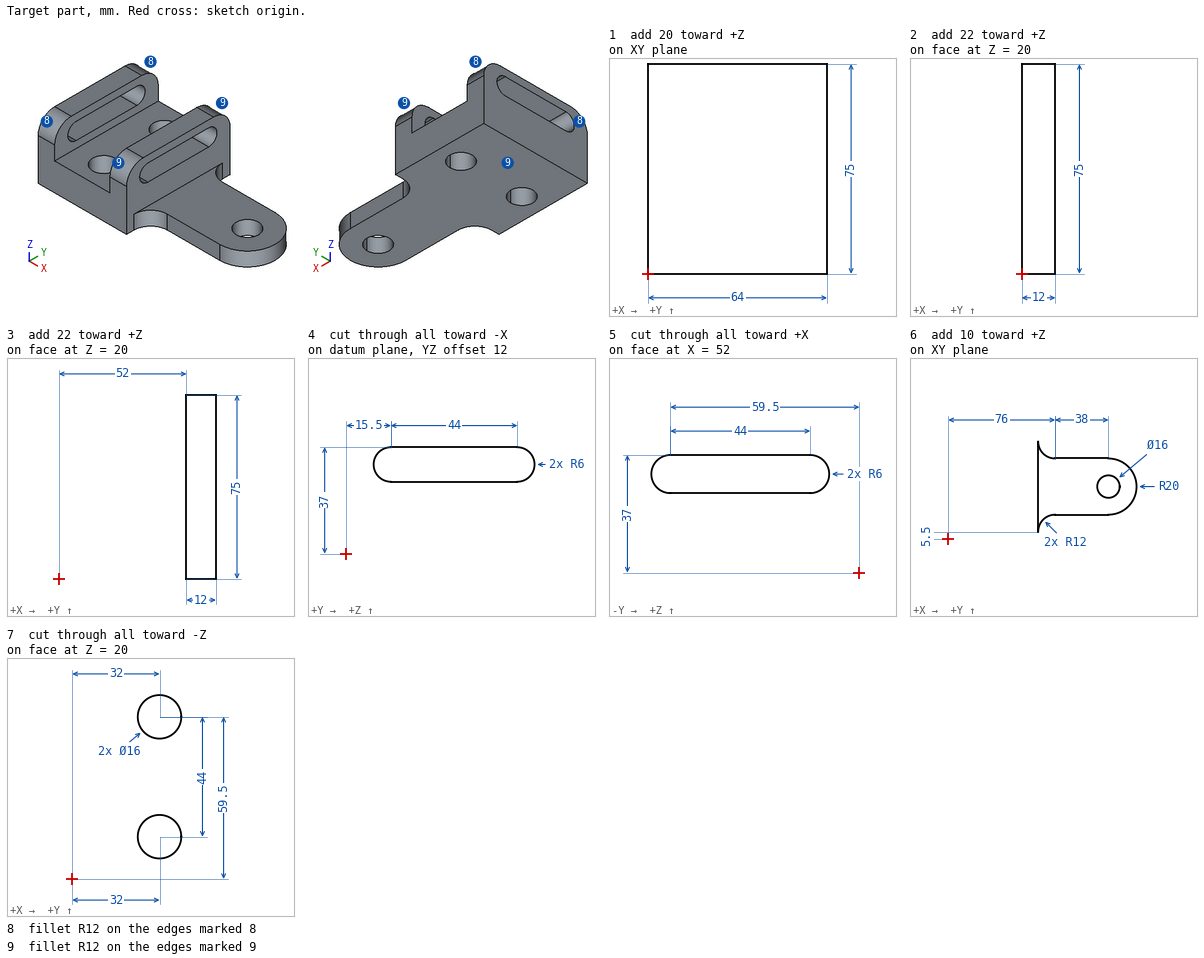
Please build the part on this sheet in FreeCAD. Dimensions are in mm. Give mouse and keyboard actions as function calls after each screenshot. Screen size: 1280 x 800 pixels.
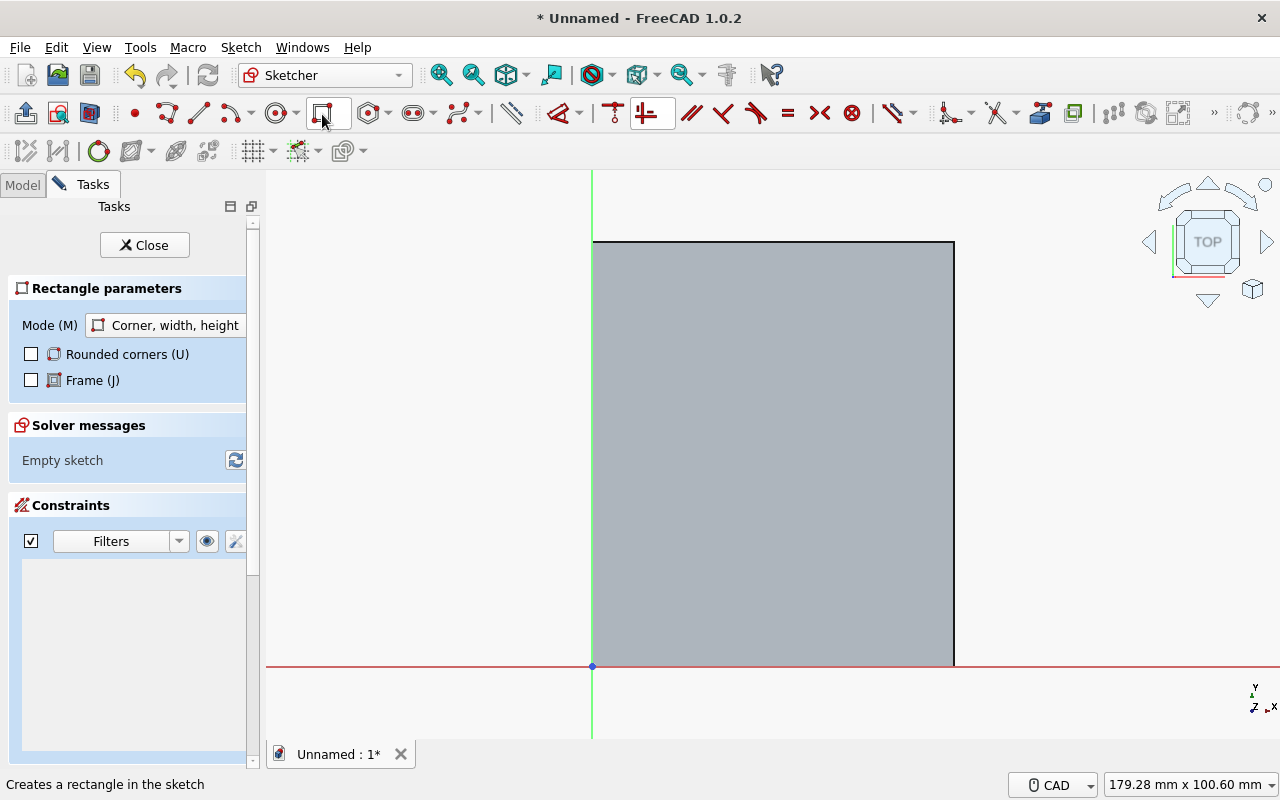
click(592, 667)
click(660, 242)
key(Escape)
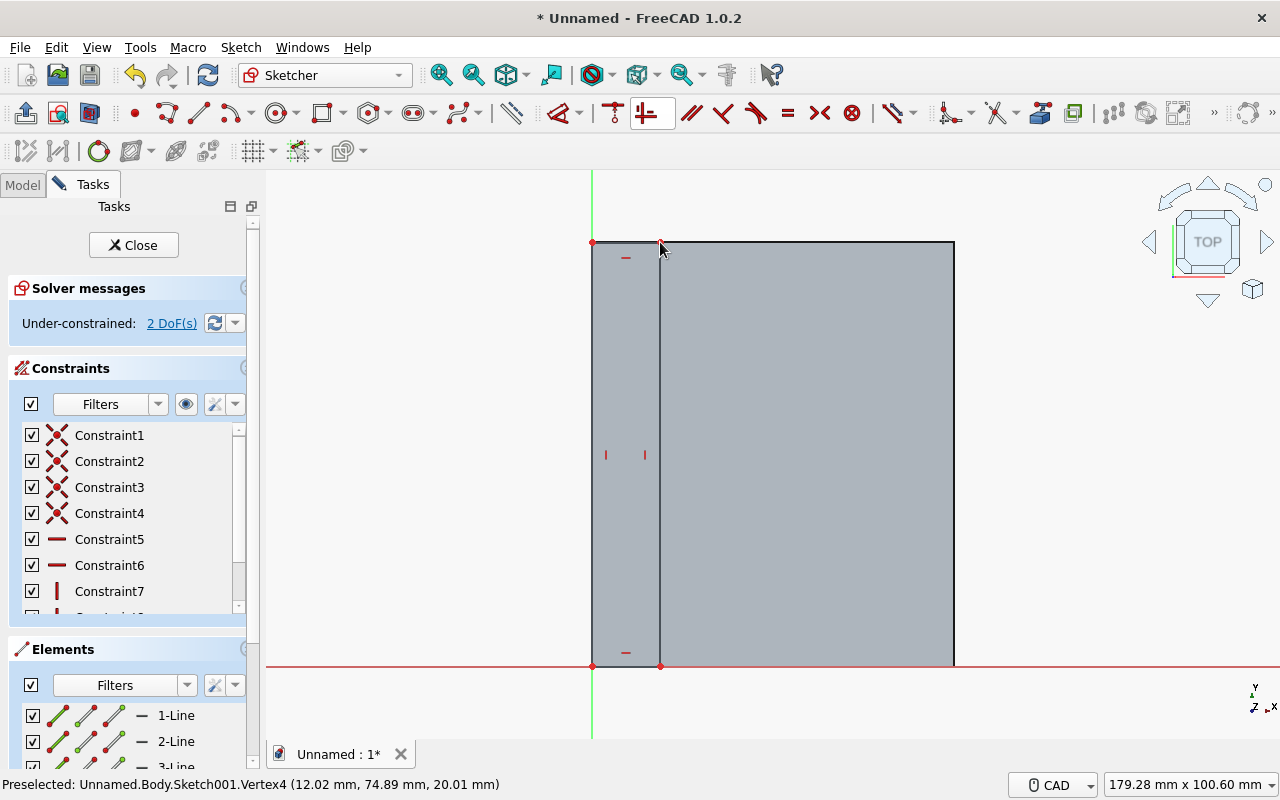
click(558, 114)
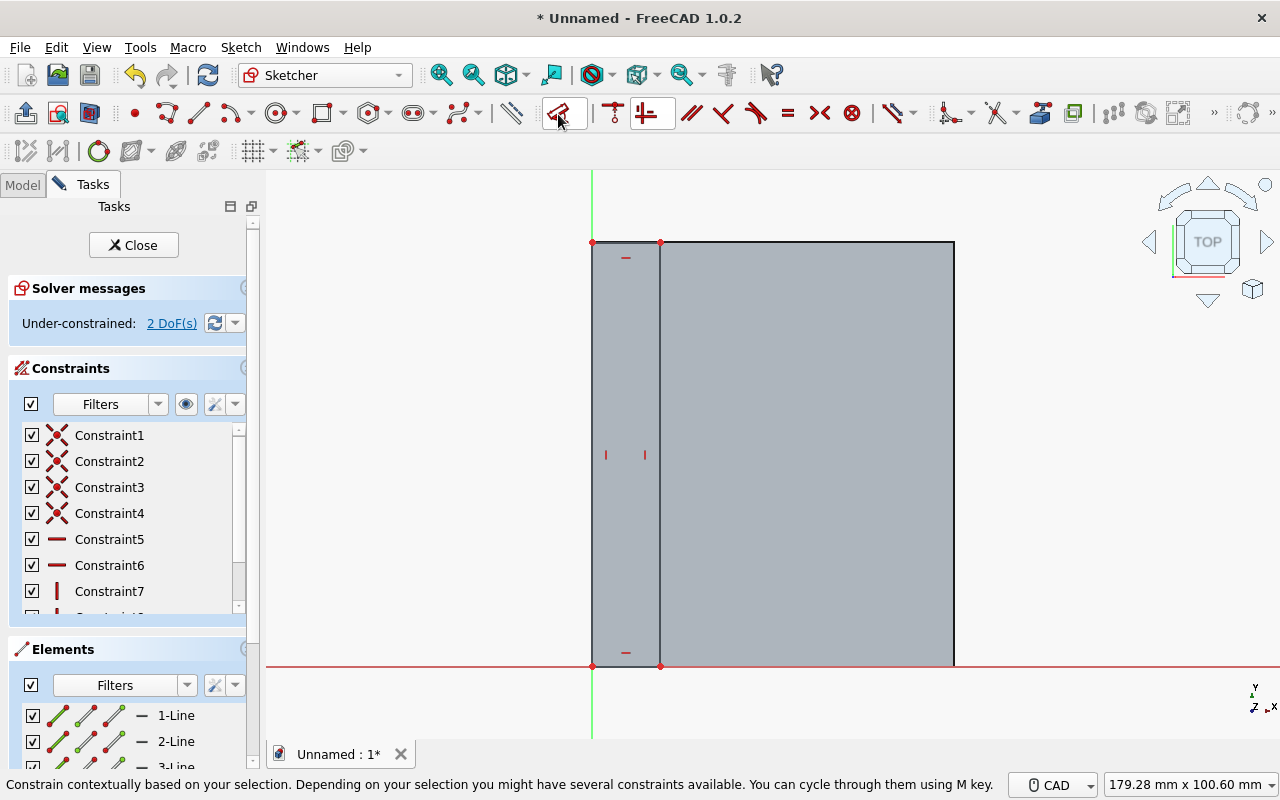
click(612, 667)
click(626, 701)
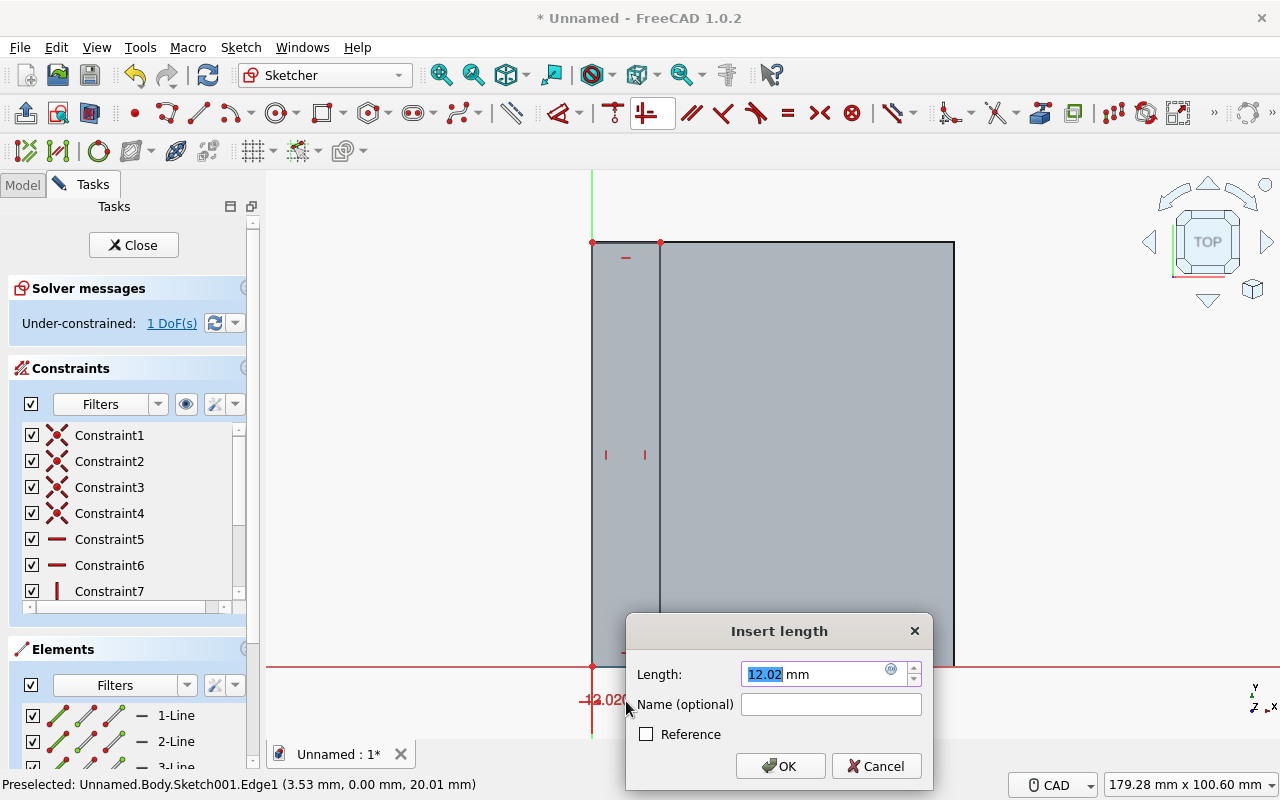
text(12)
key(Return)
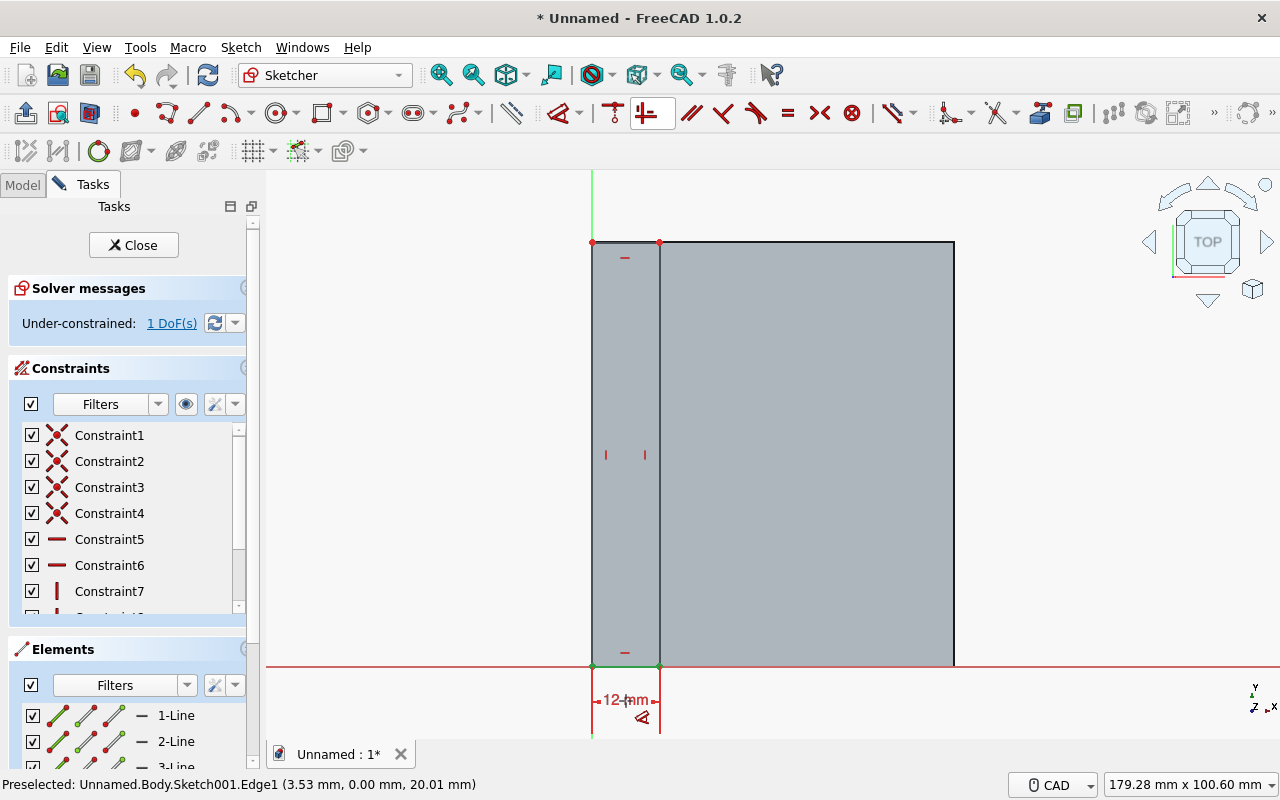
click(660, 540)
click(694, 455)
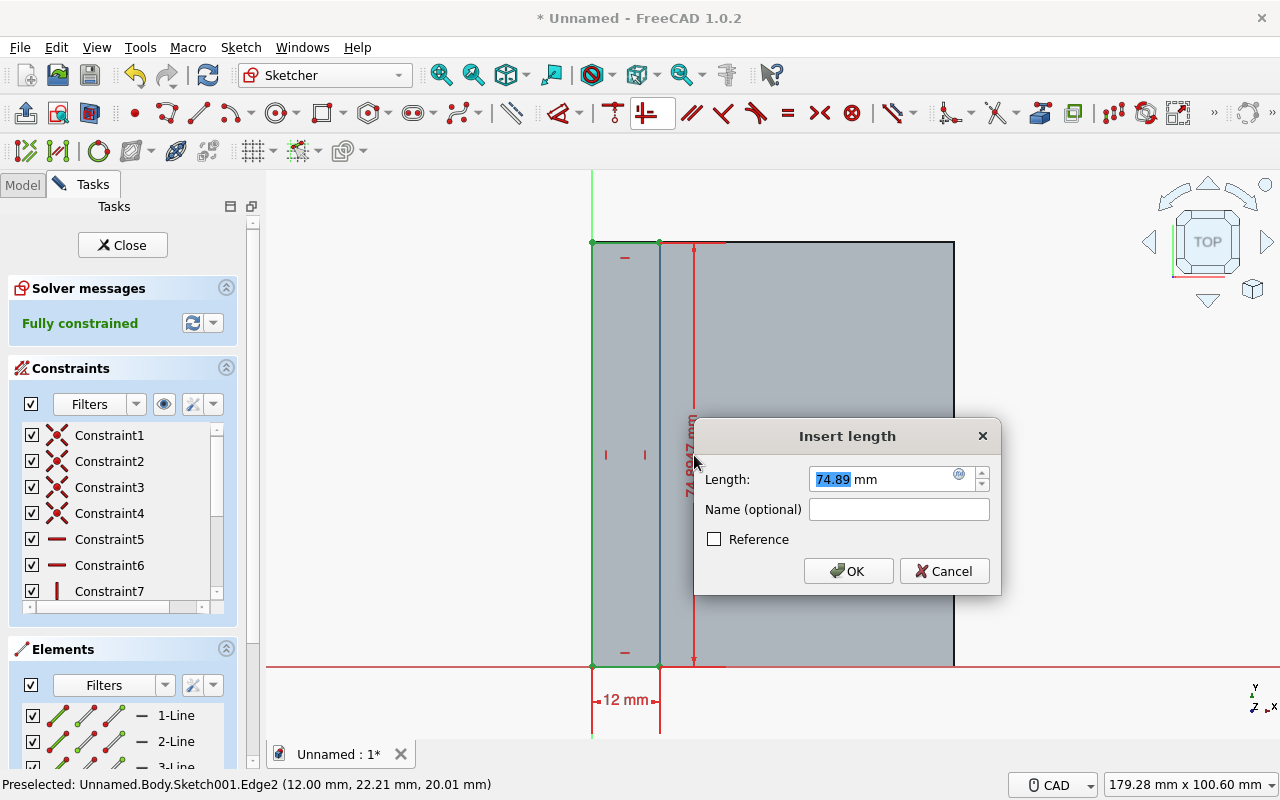
text(75)
key(Return)
key(Escape)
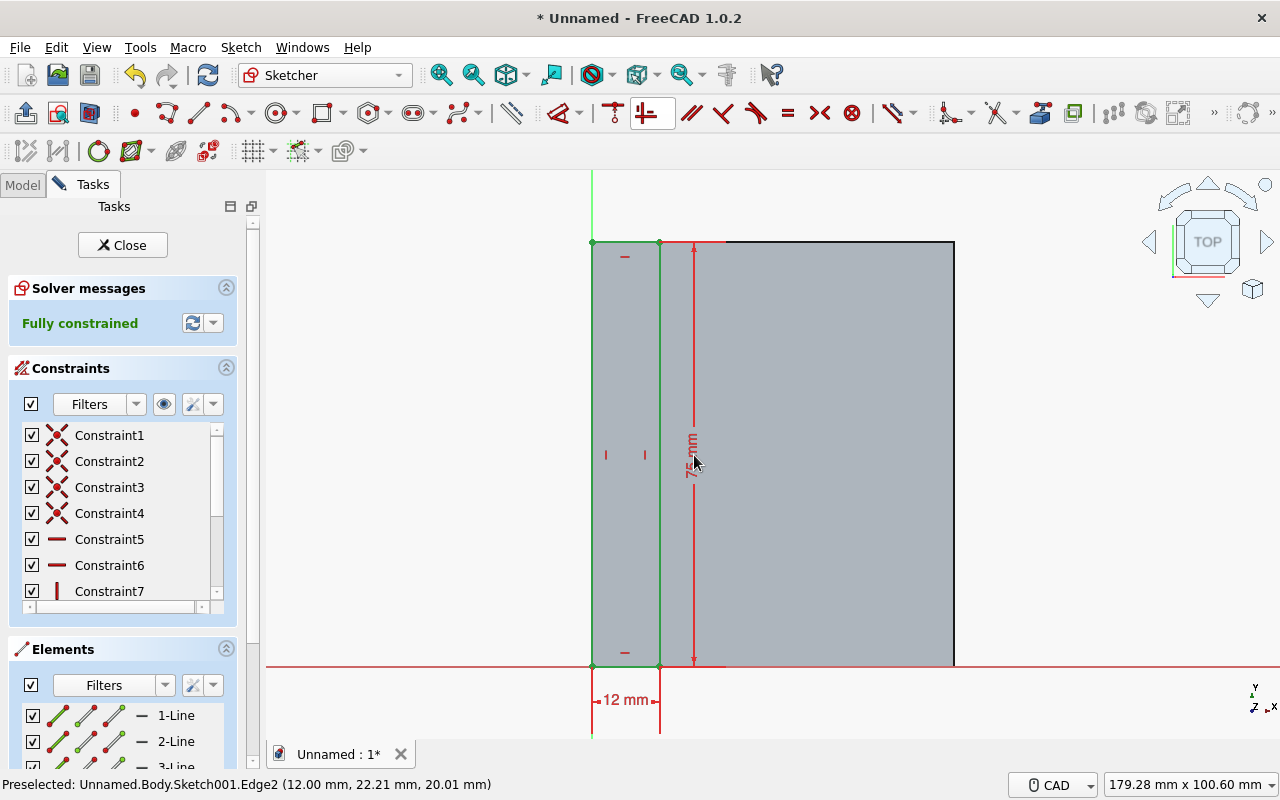
click(123, 245)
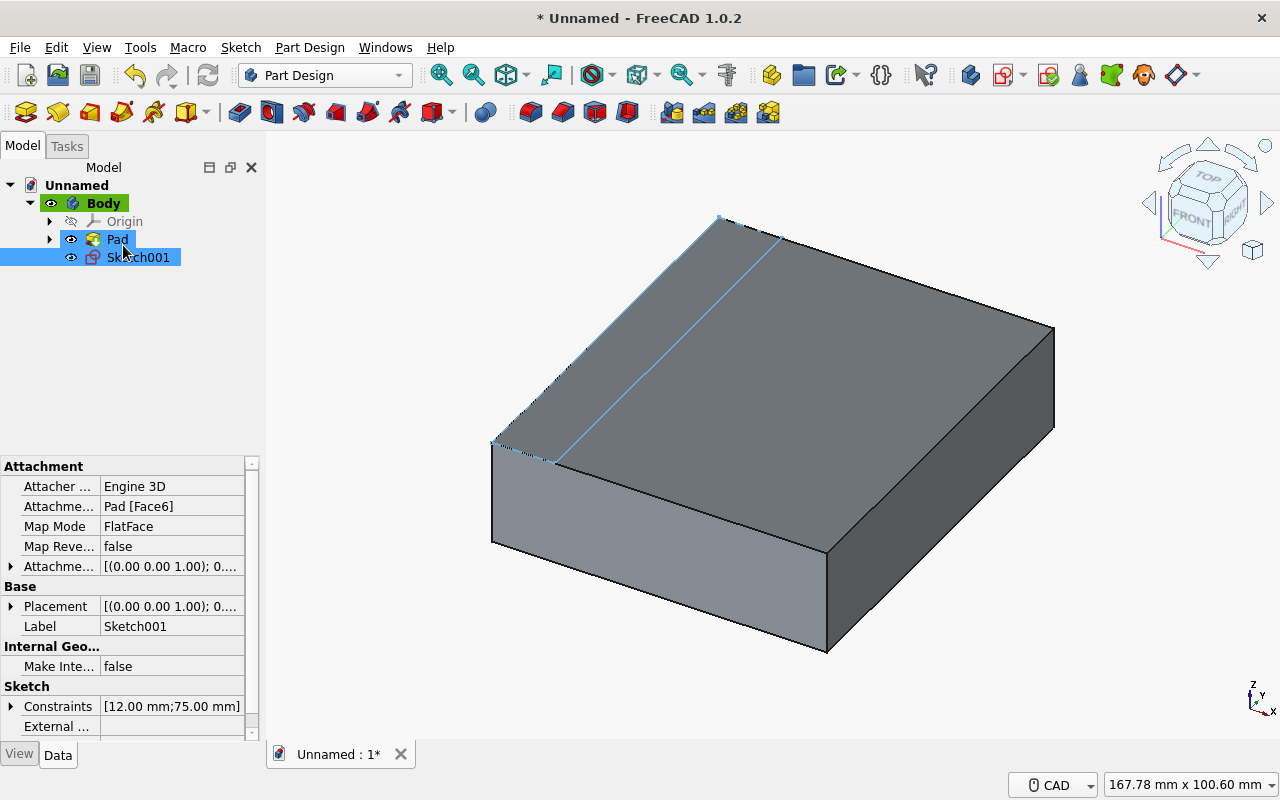
click(26, 112)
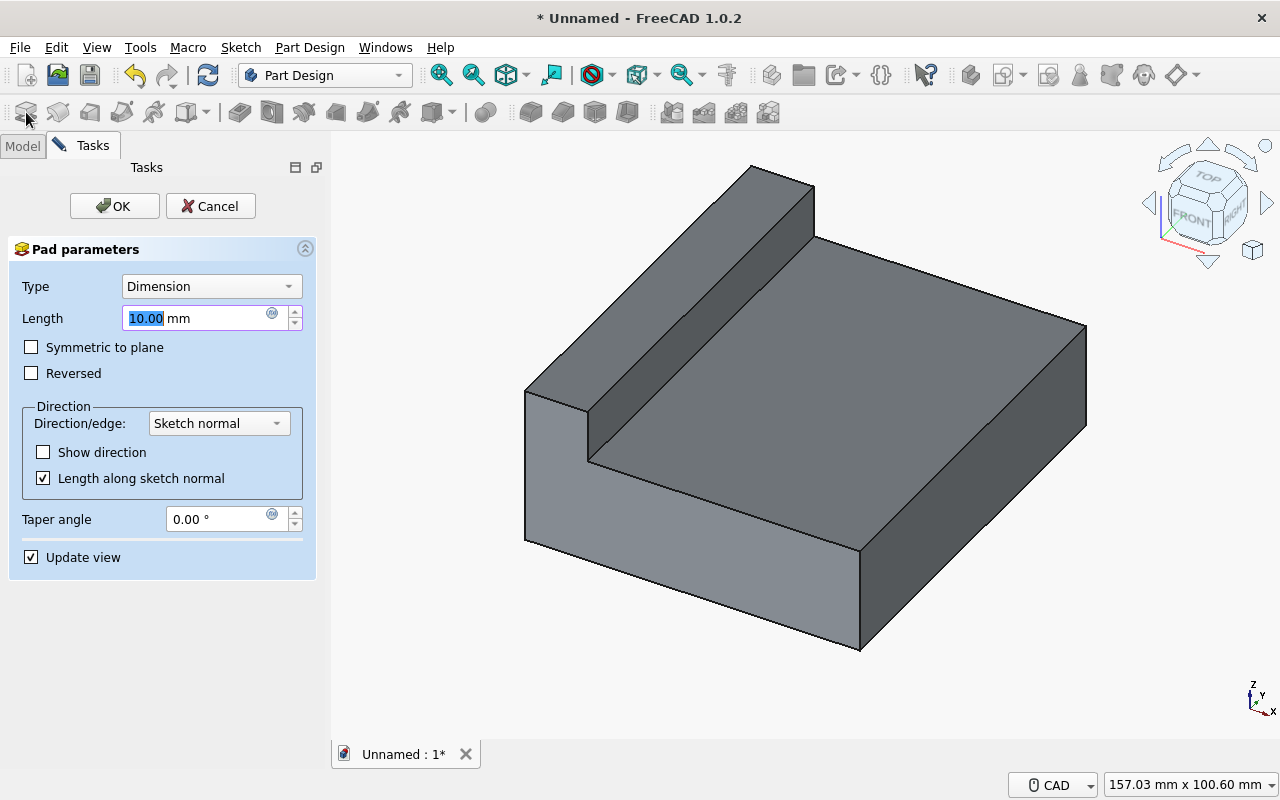
text(22)
key(Tab)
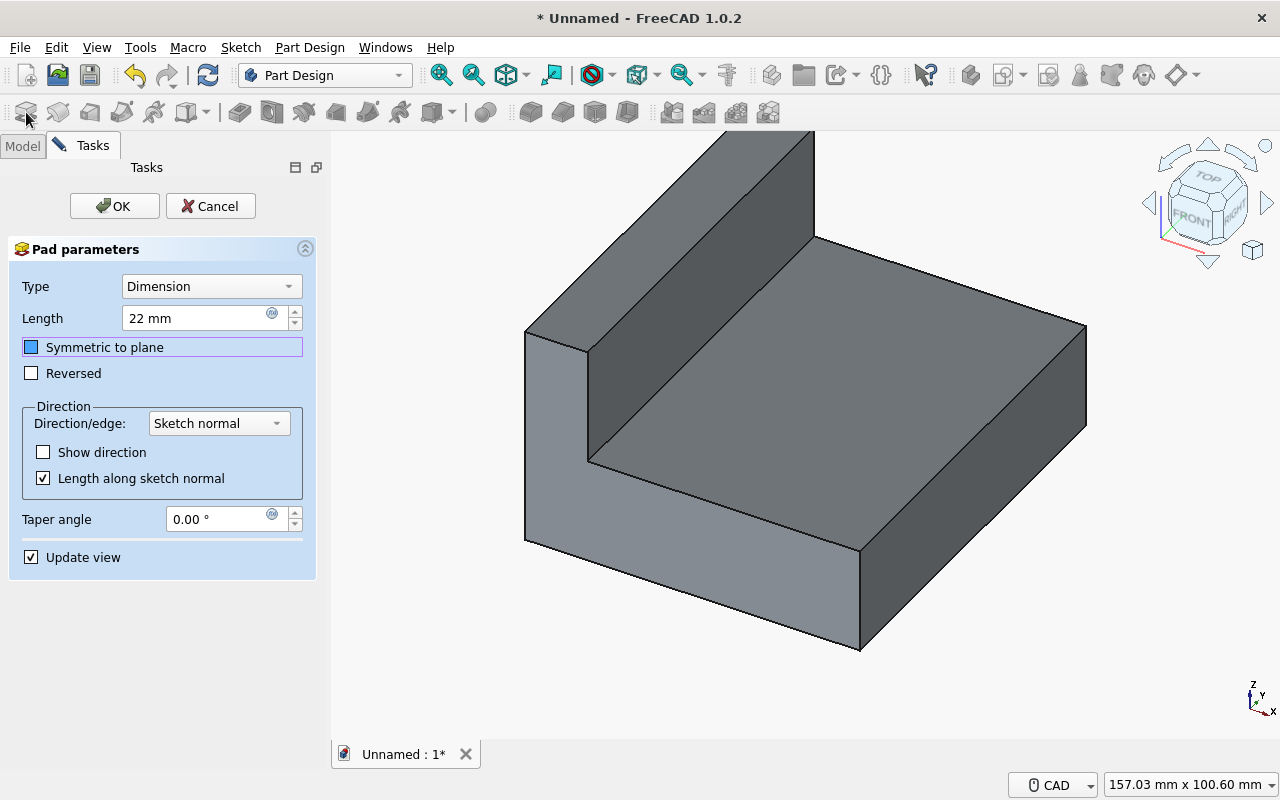
click(115, 206)